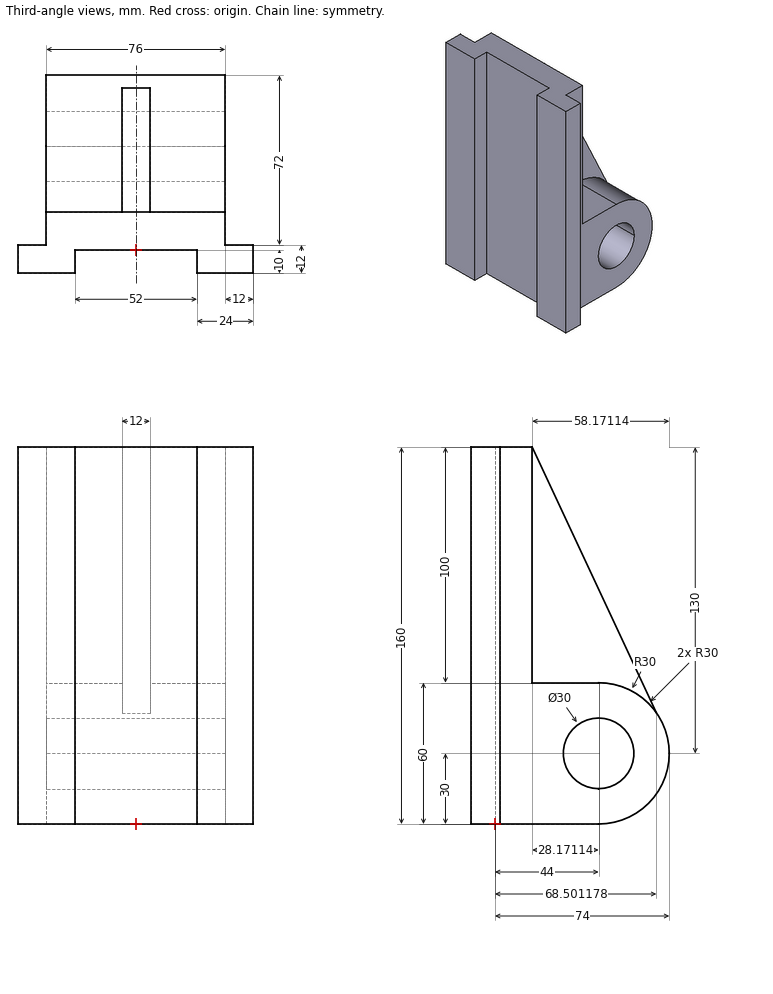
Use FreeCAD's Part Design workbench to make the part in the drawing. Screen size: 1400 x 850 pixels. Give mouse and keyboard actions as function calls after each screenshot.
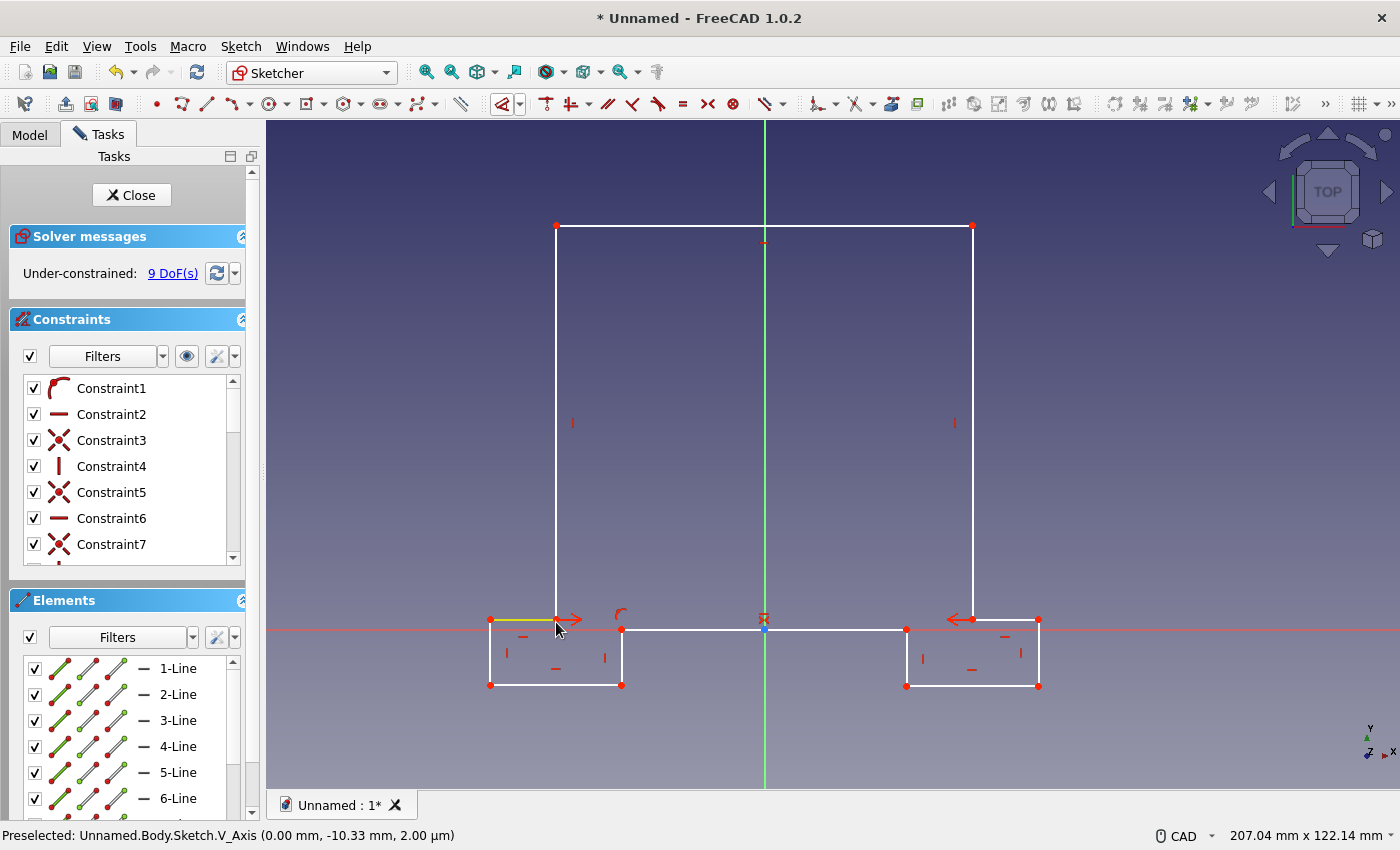
click(1039, 686)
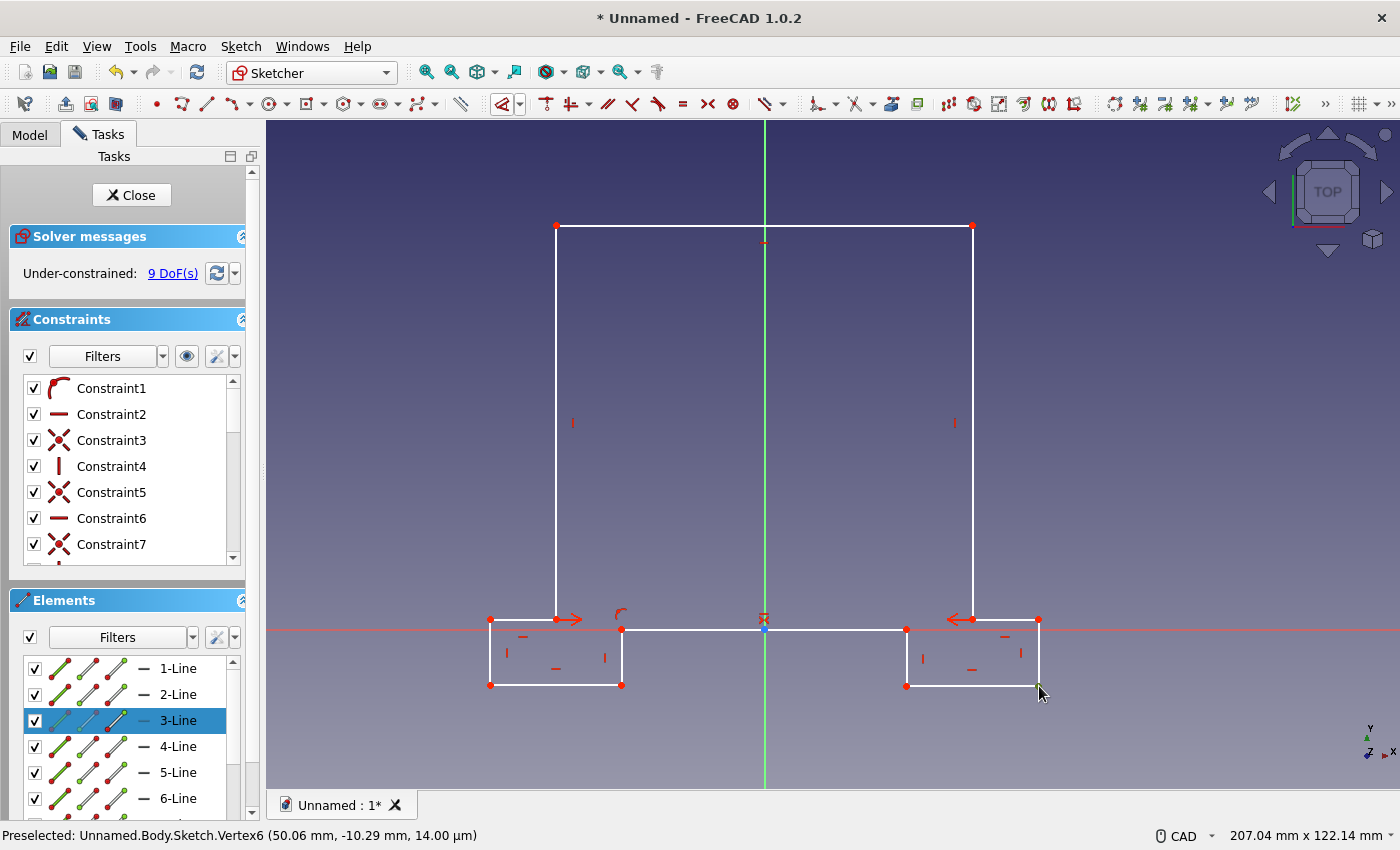
click(490, 685)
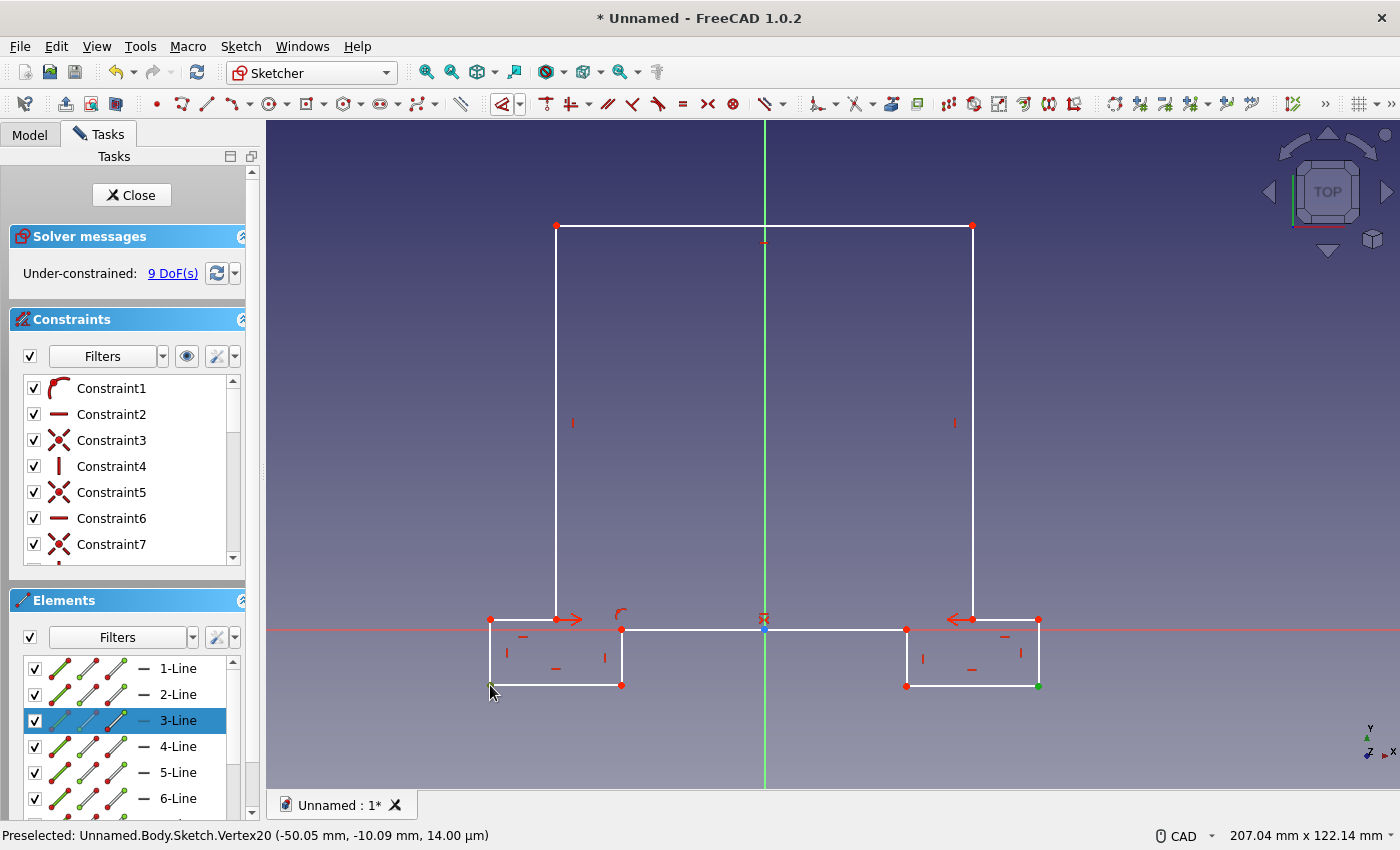
click(765, 717)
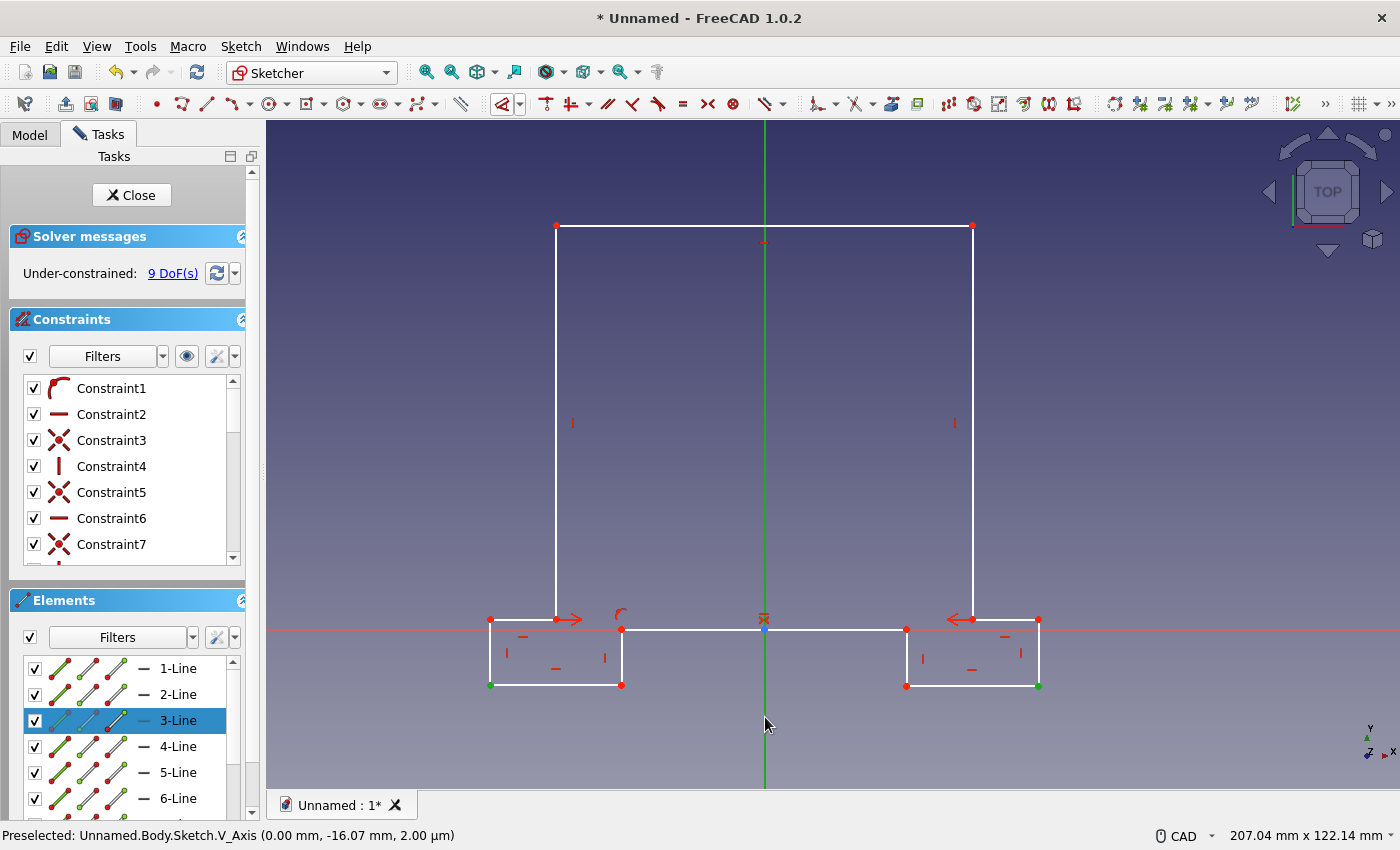
click(708, 104)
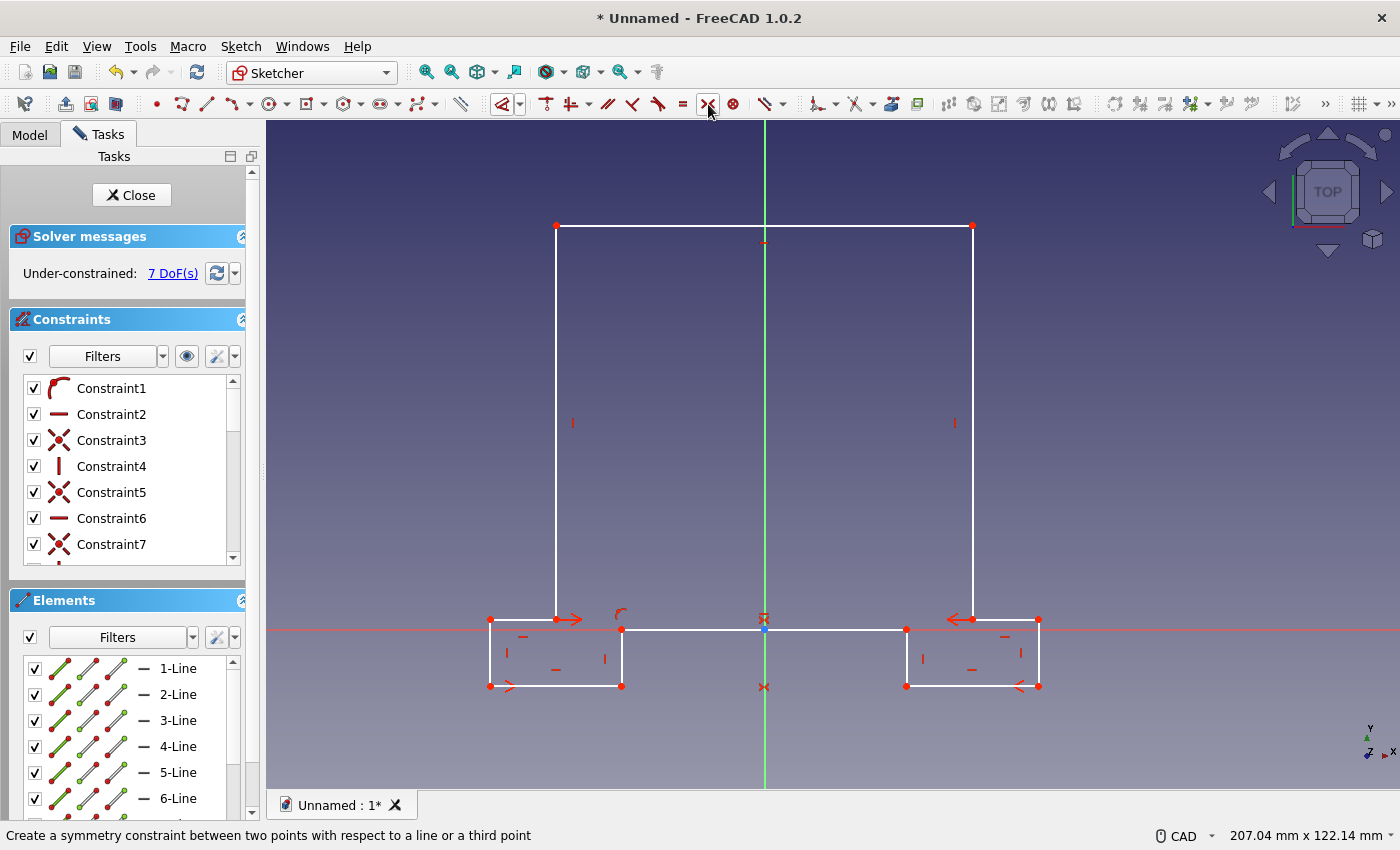
key(d)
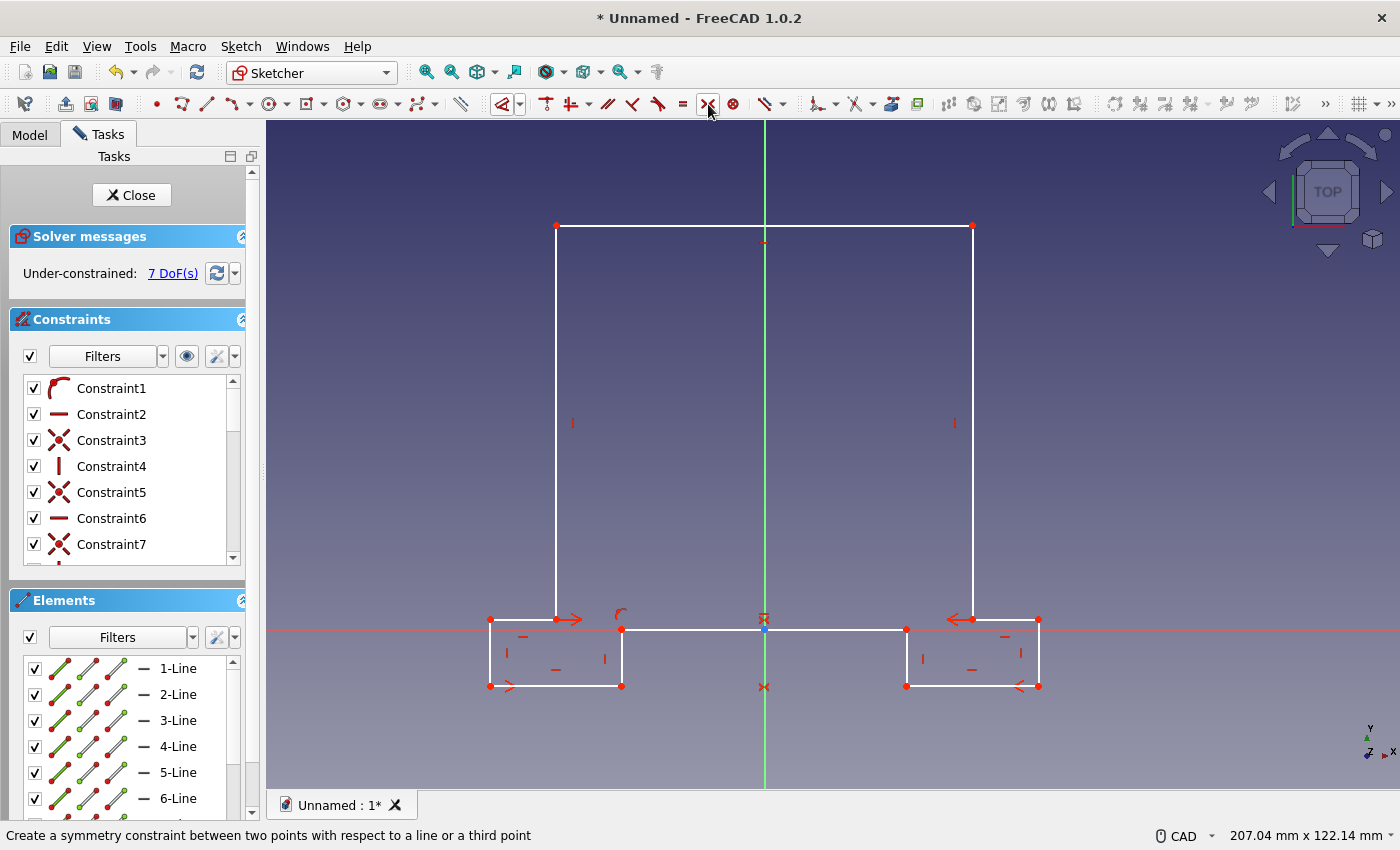
click(707, 630)
click(699, 664)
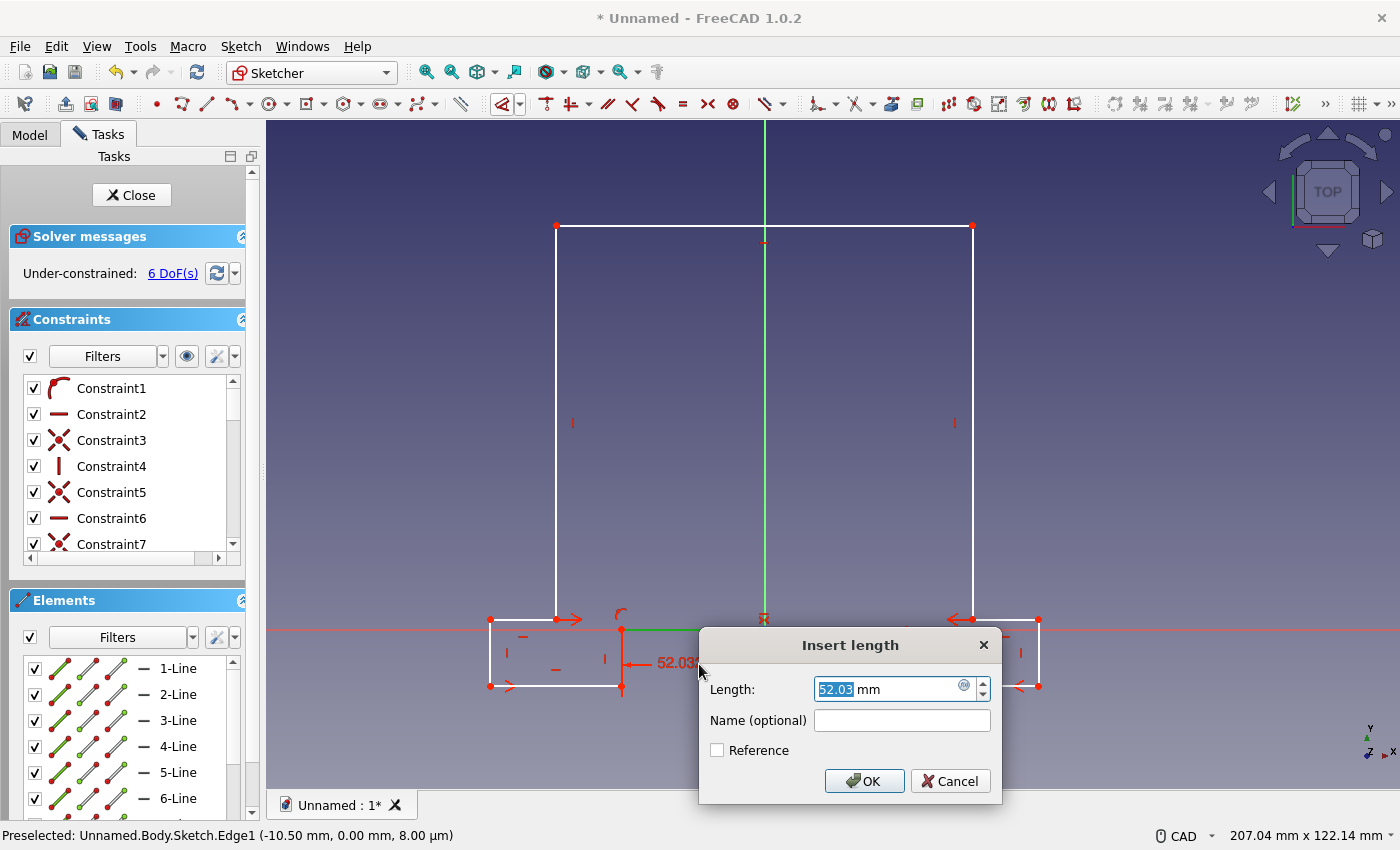
text(52)
key(Return)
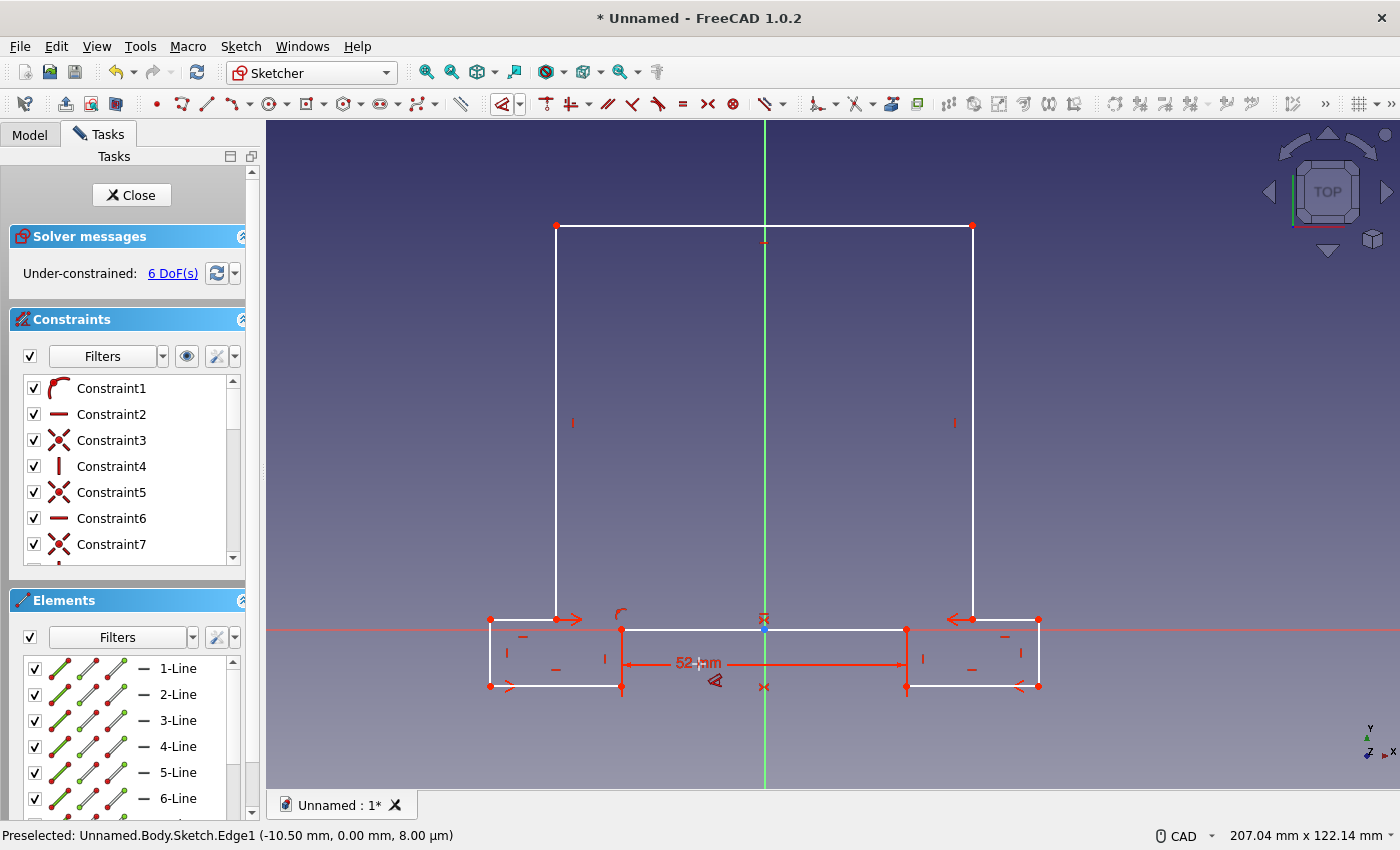
click(907, 647)
click(941, 658)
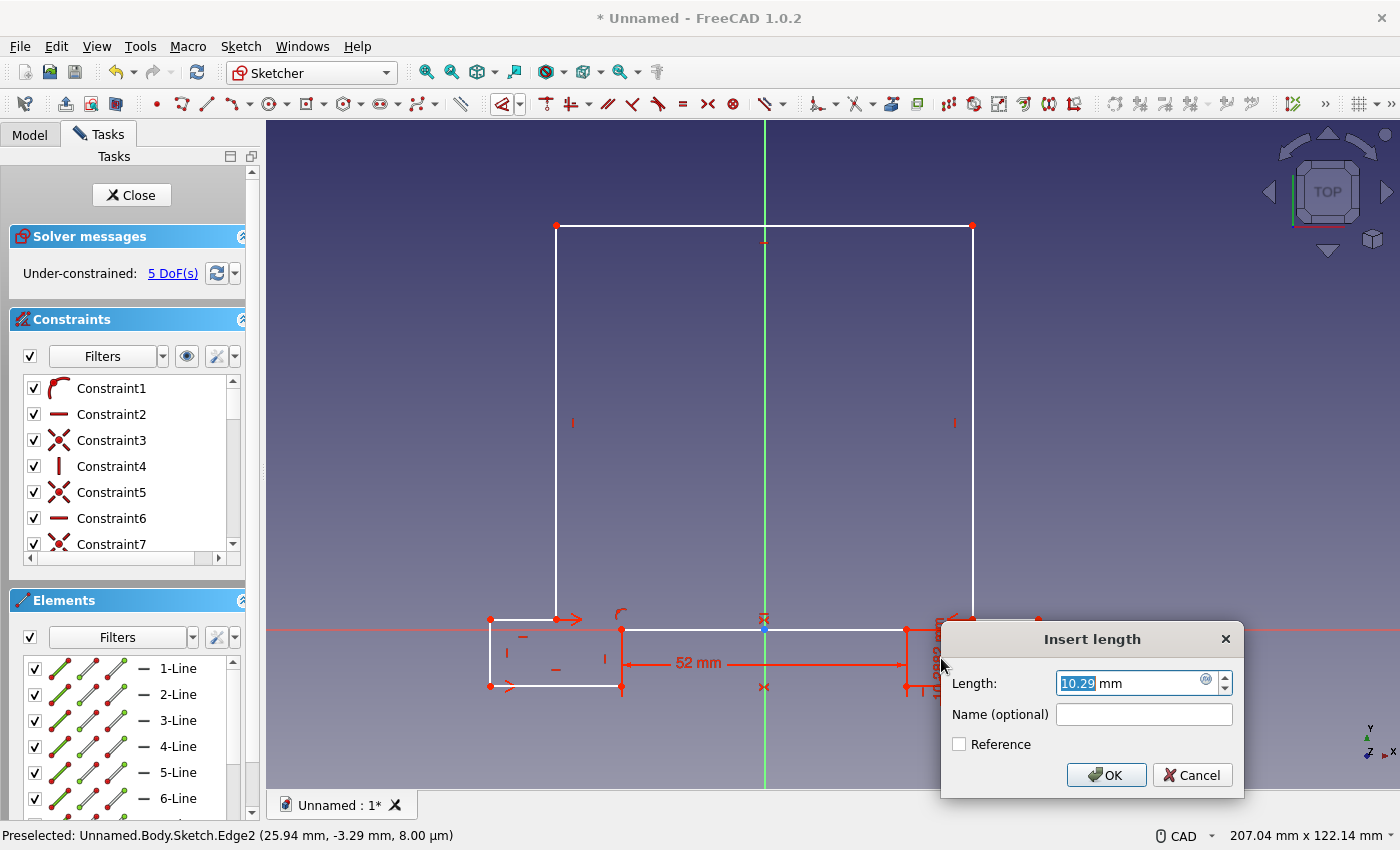
text(10)
key(Return)